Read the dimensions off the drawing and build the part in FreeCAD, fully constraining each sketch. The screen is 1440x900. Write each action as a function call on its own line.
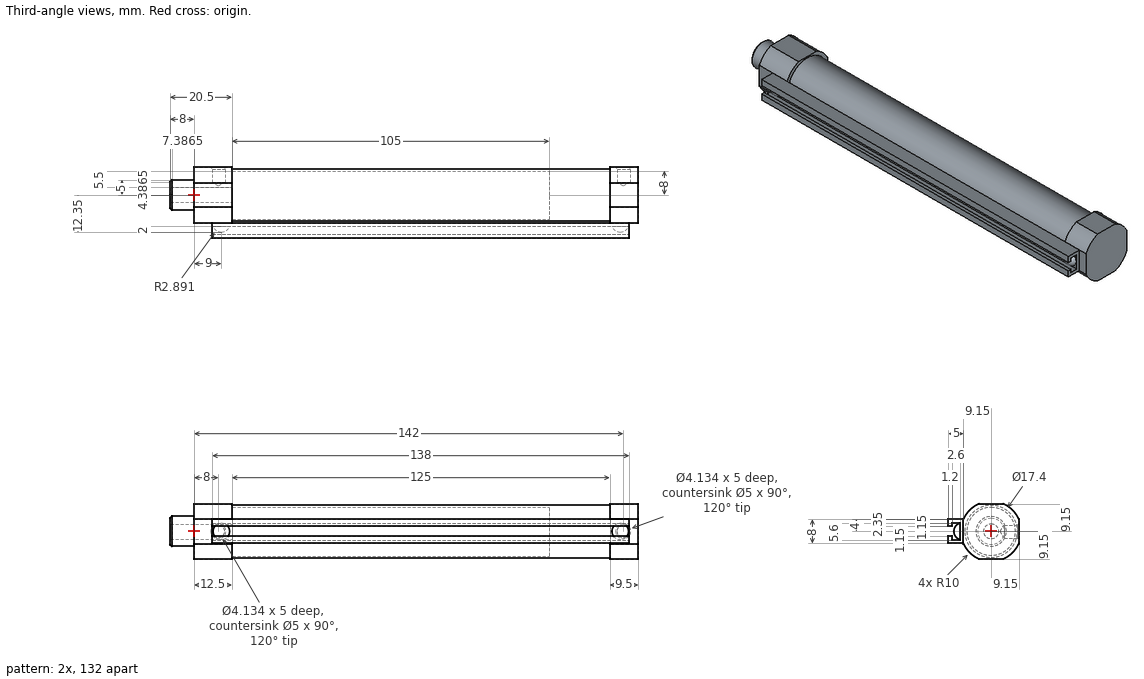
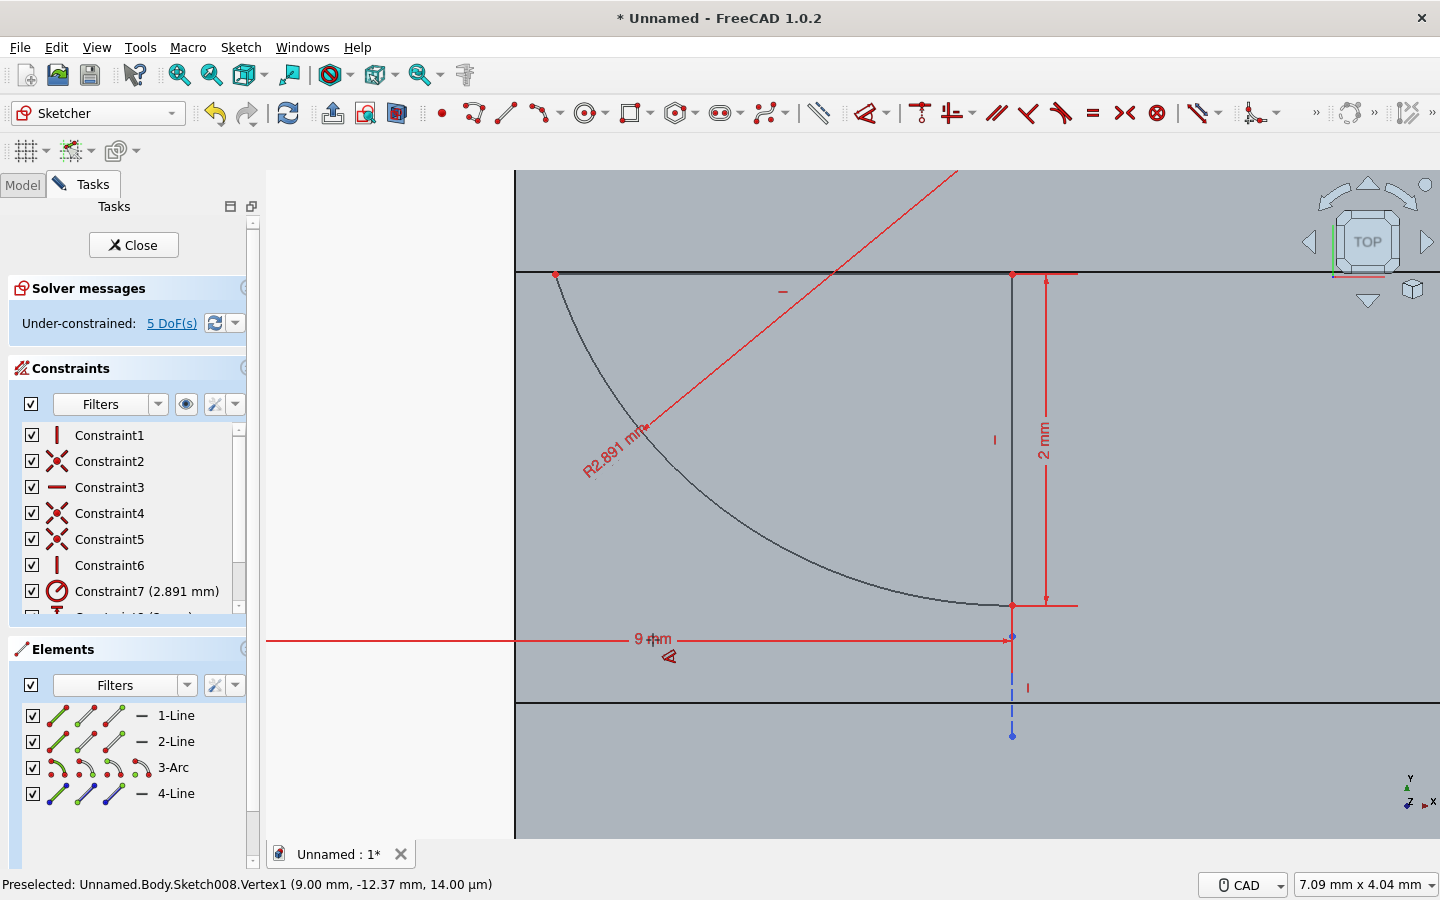
click(1012, 637)
click(653, 671)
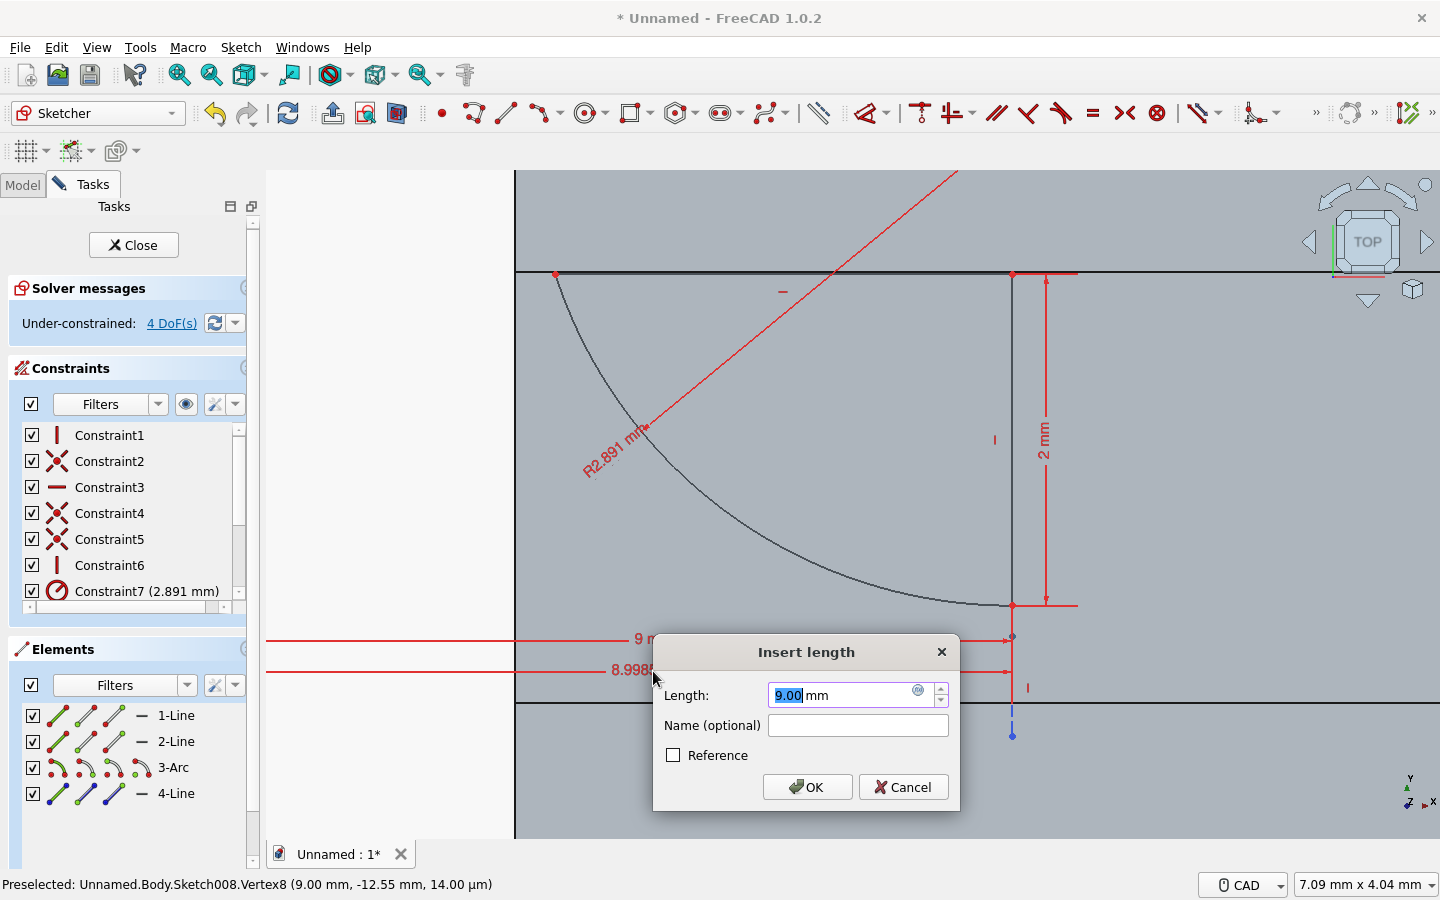
text(9)
key(Return)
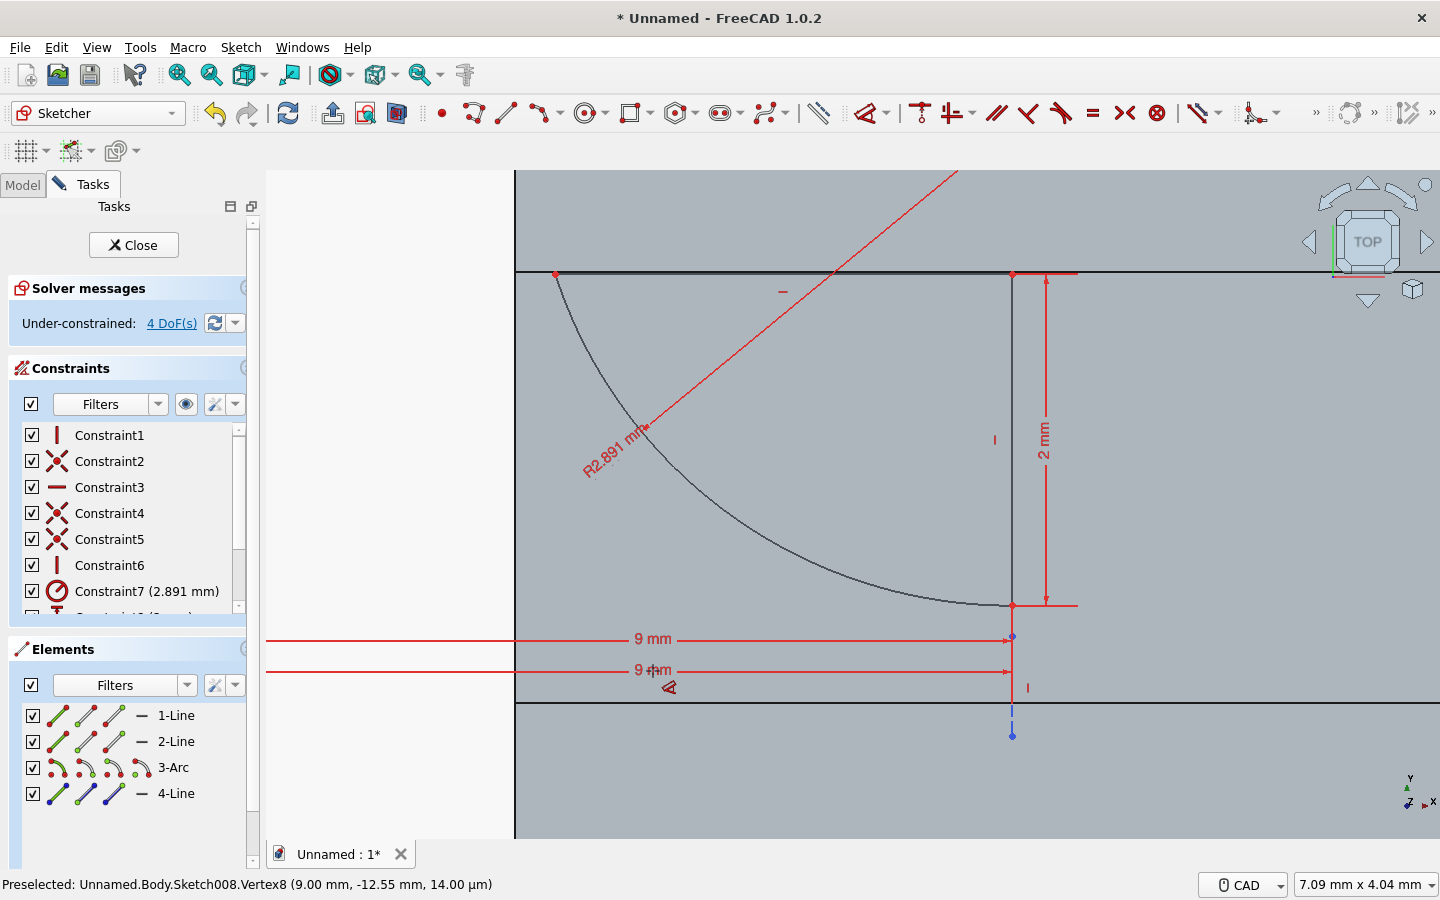
scroll(785, 654, down, 2)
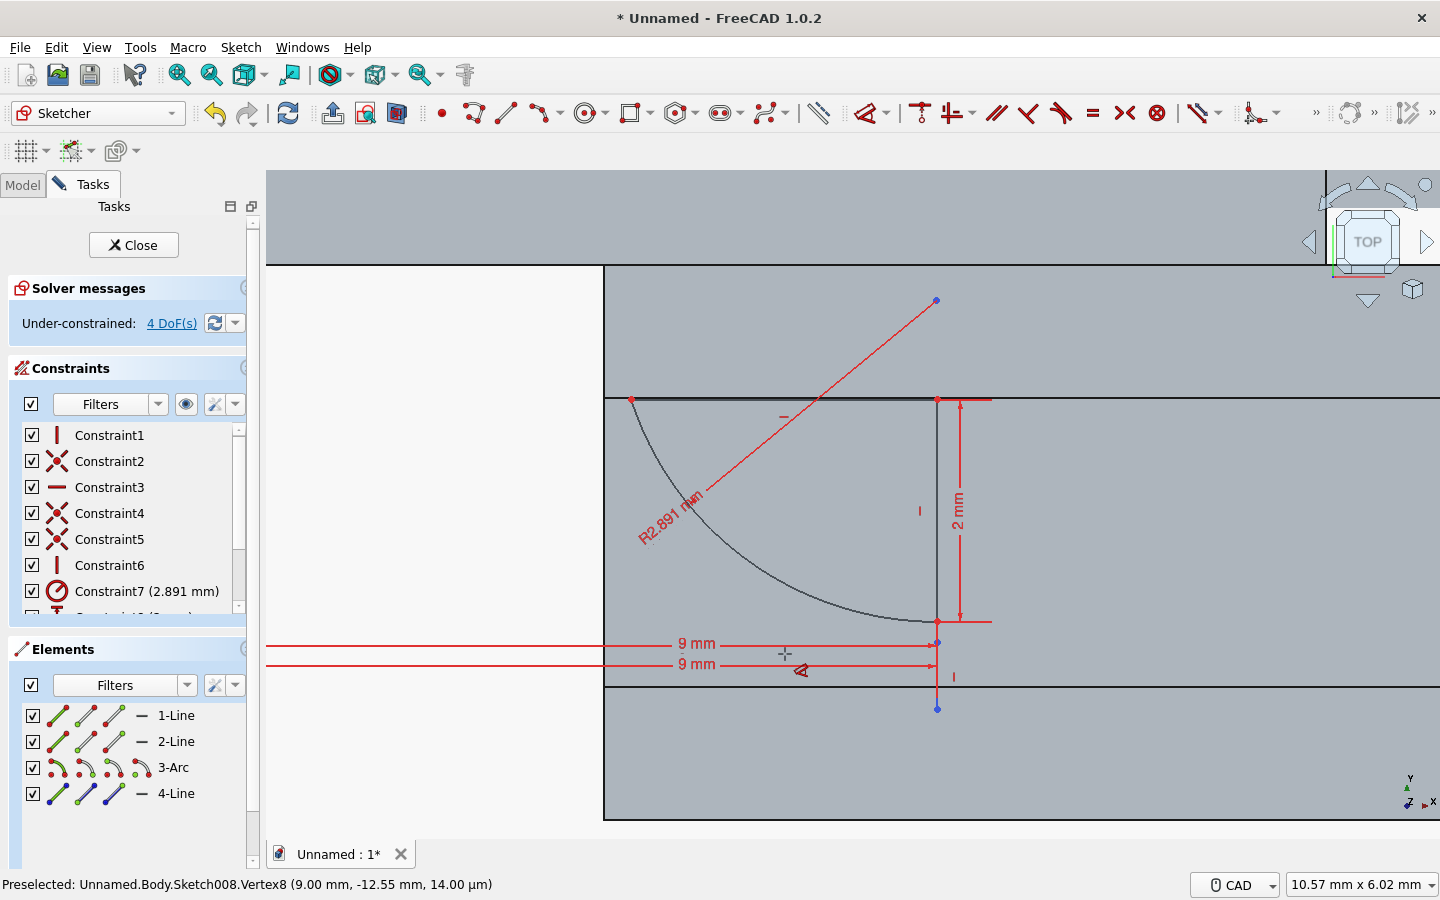
click(937, 301)
click(615, 335)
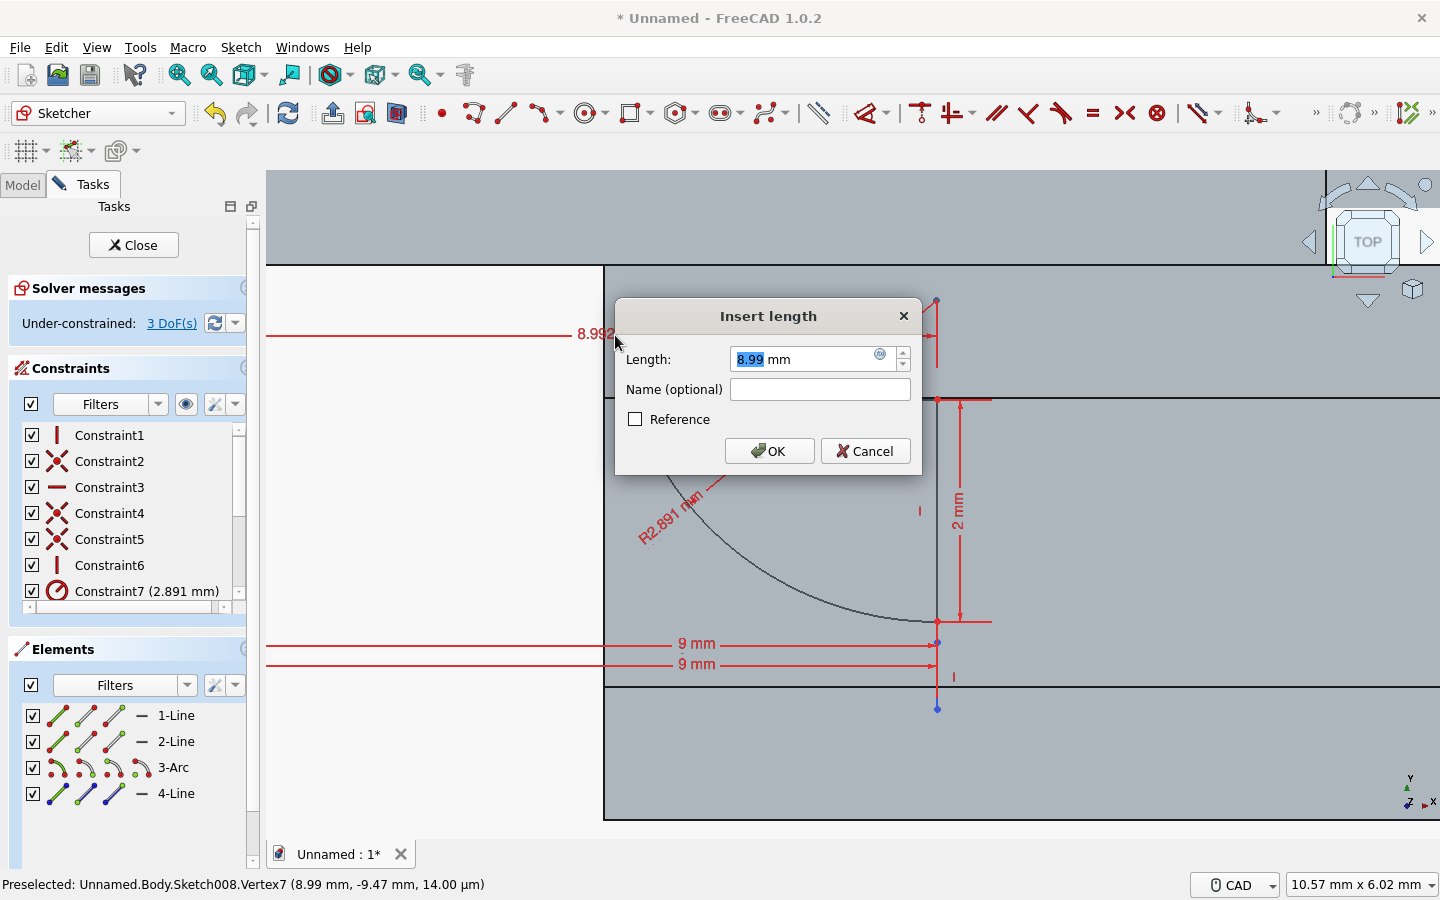
text(9)
key(Return)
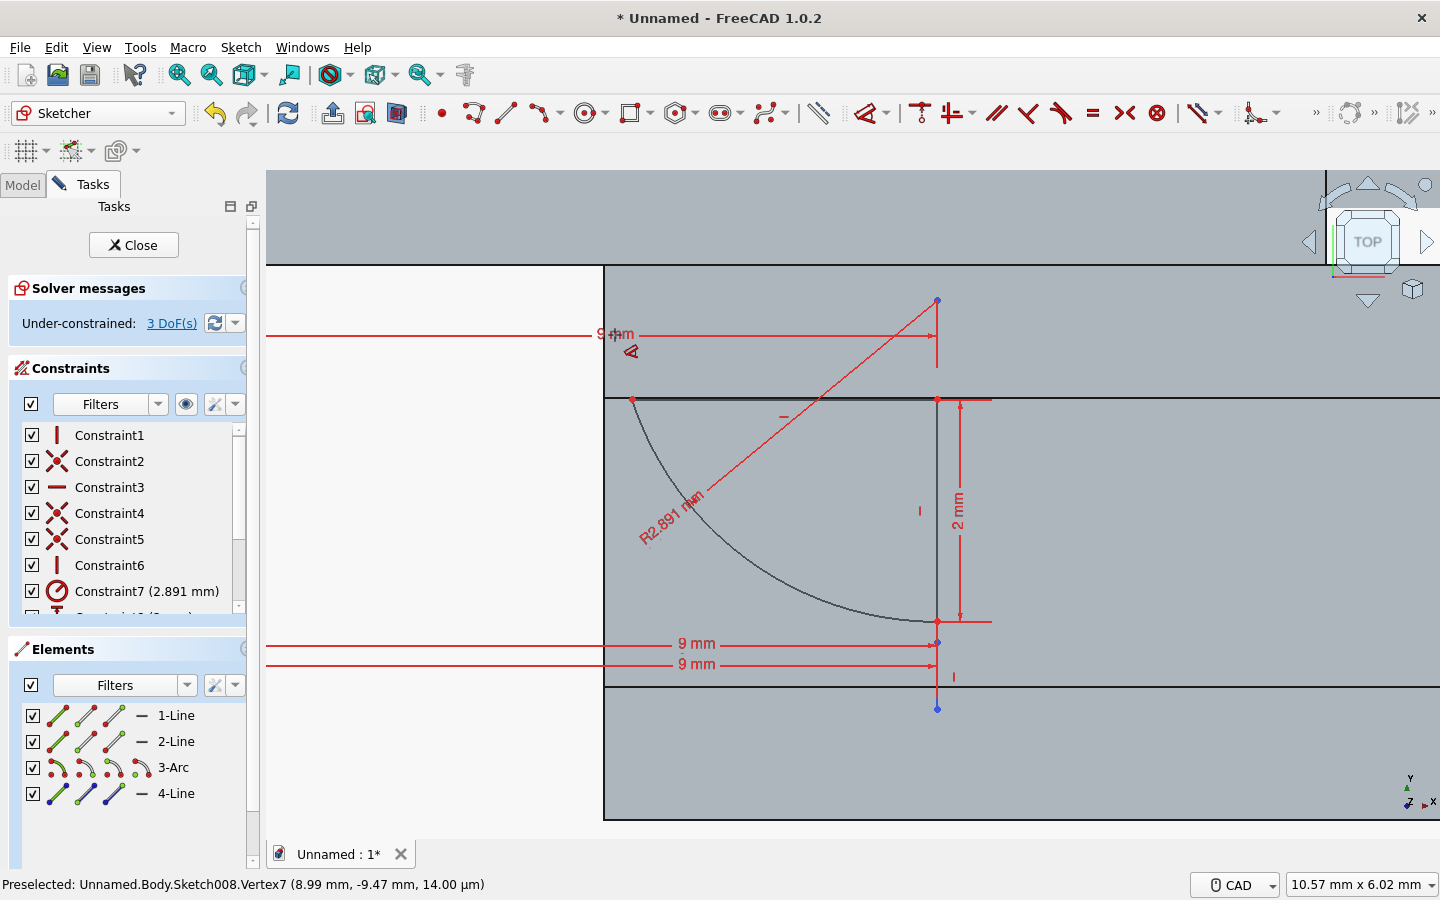
click(937, 622)
click(971, 410)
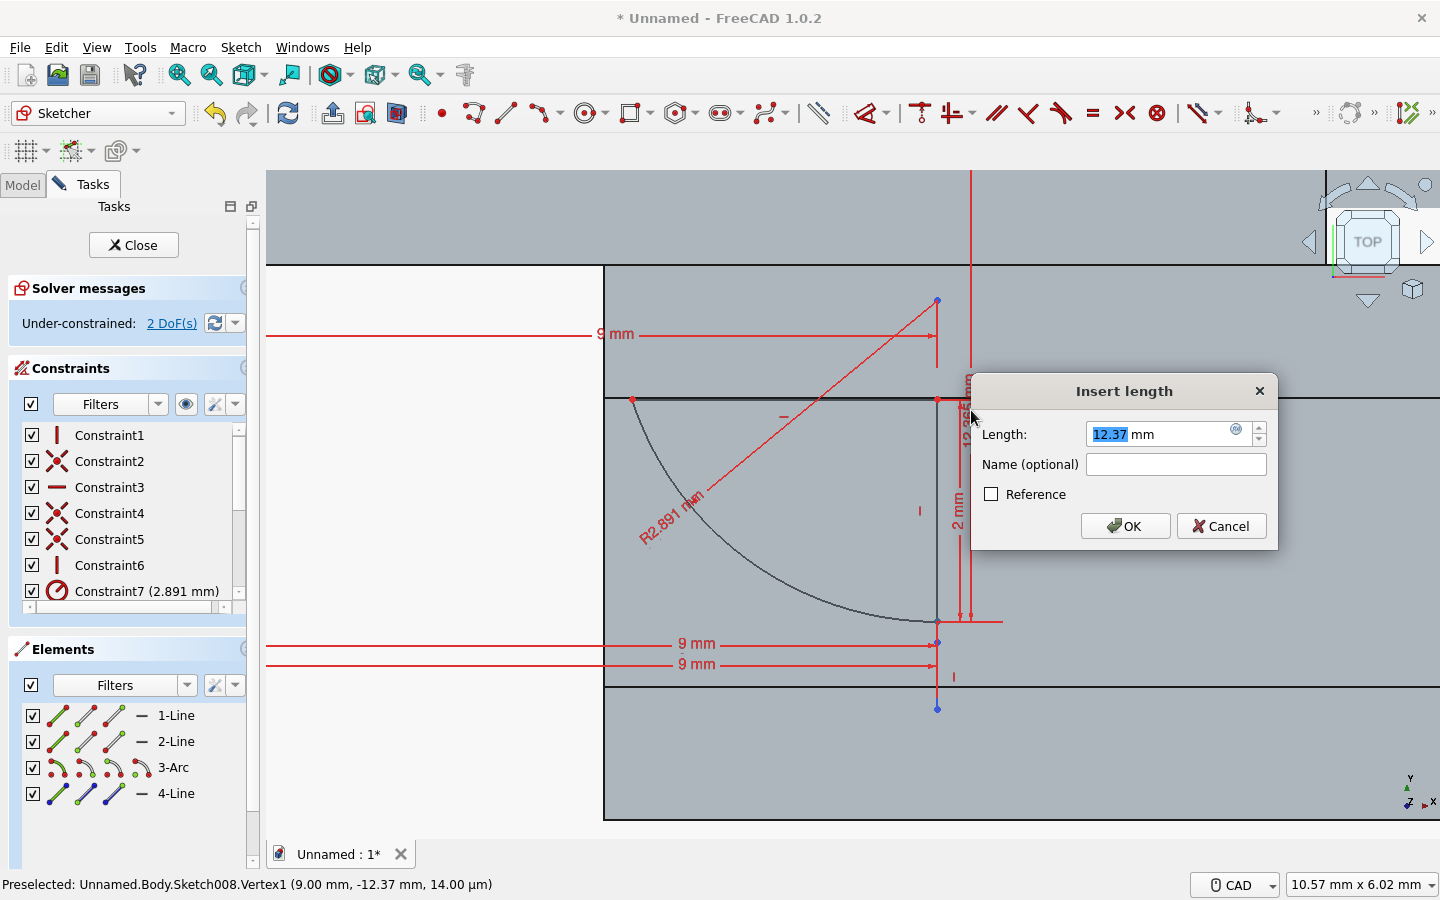
text(12.35)
key(Return)
key(Escape)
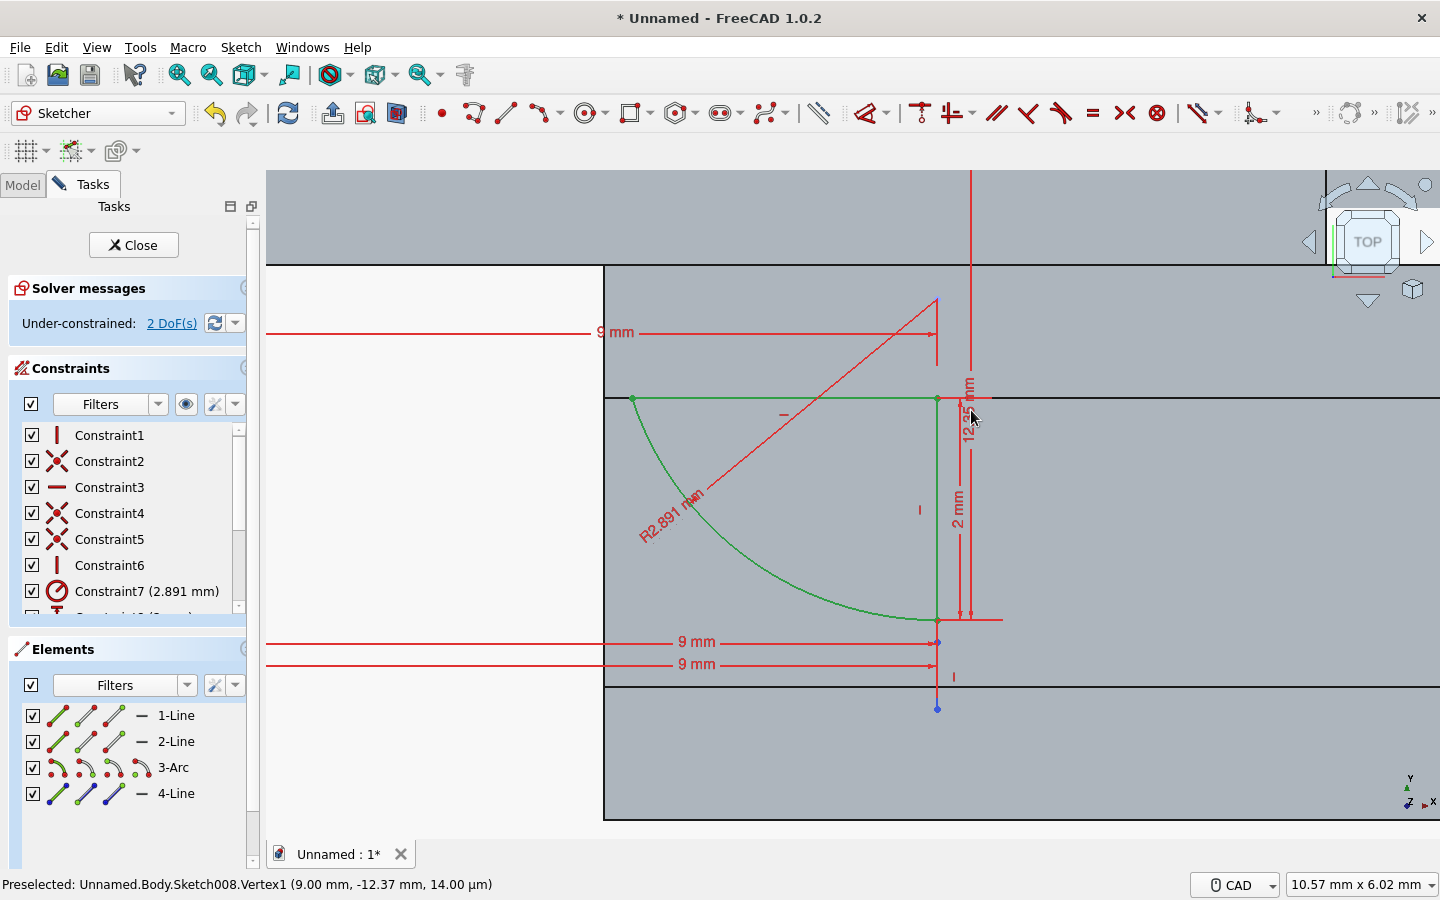
click(134, 245)